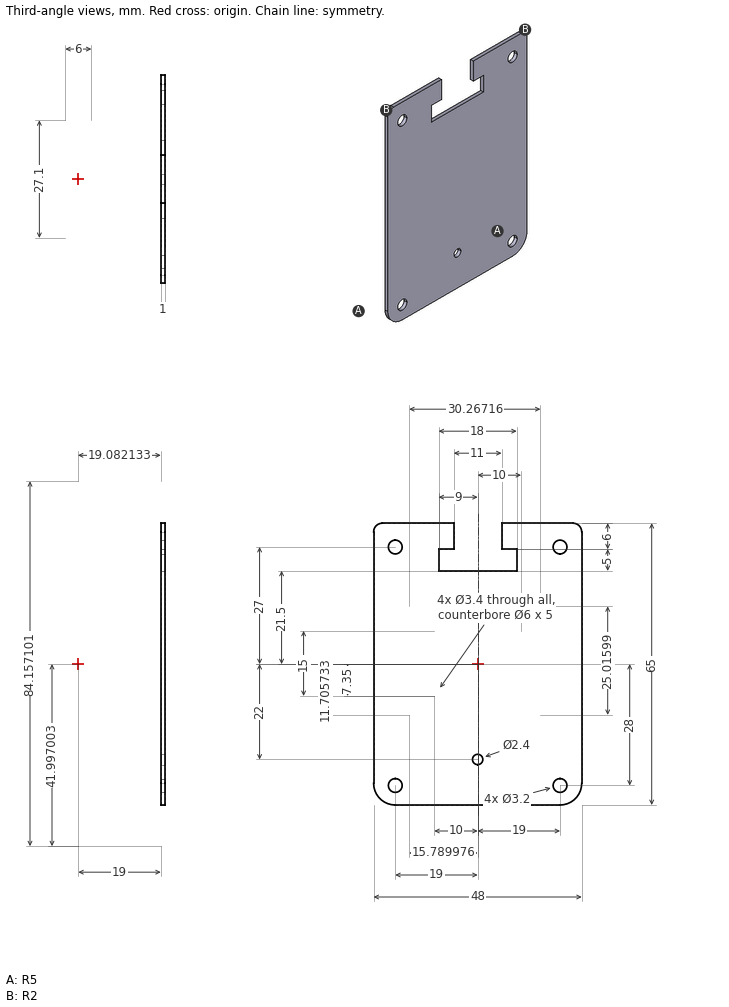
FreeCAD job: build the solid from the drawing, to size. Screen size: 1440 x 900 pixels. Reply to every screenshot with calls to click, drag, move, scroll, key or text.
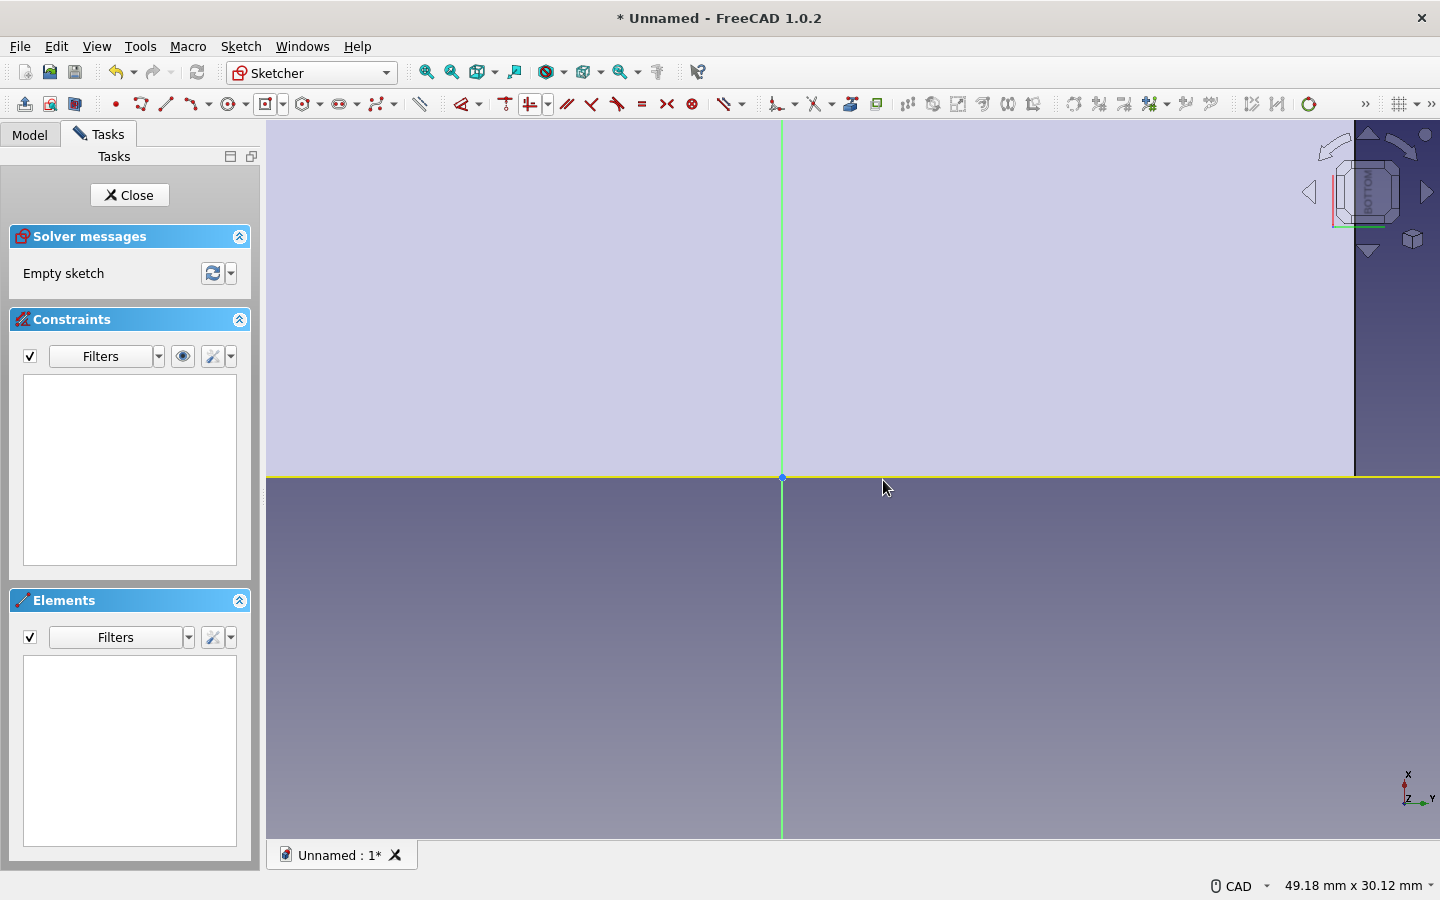
click(264, 104)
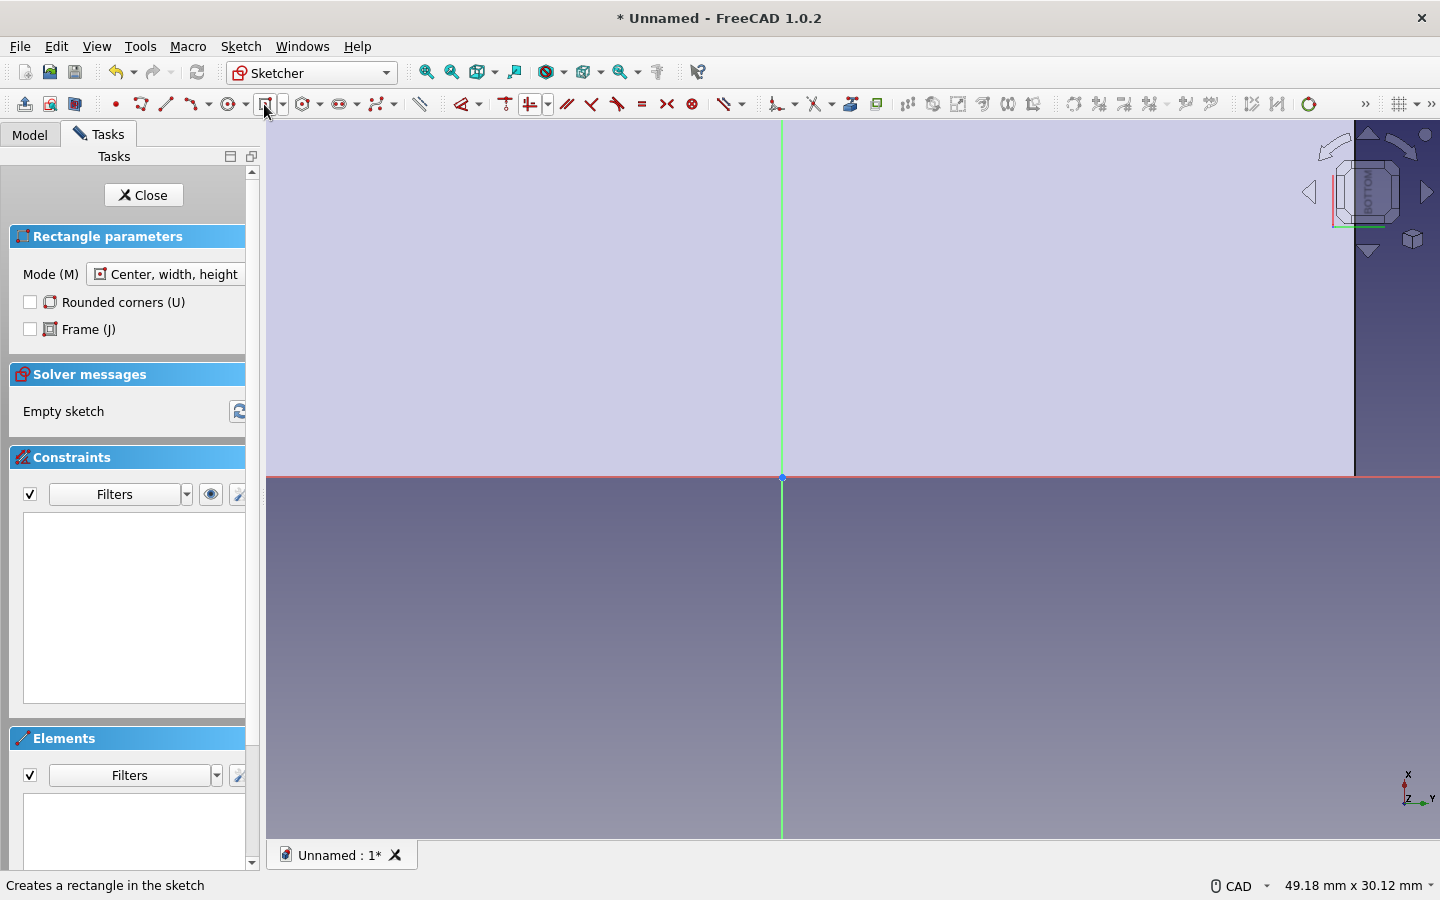
click(782, 477)
move(1106, 406)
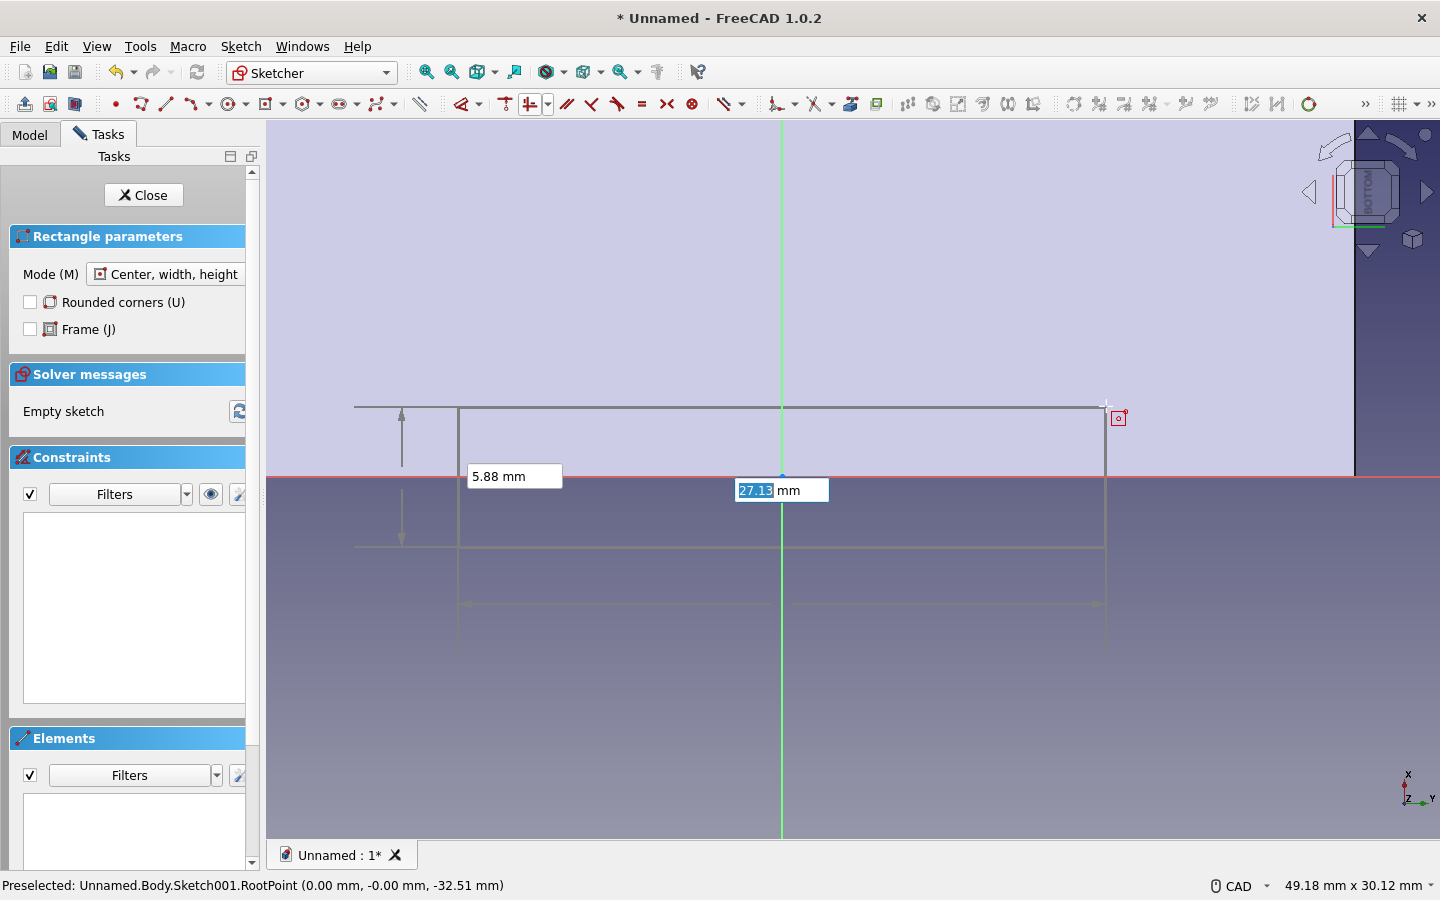
text(27.1)
key(Tab)
text(6)
key(Return)
key(Escape)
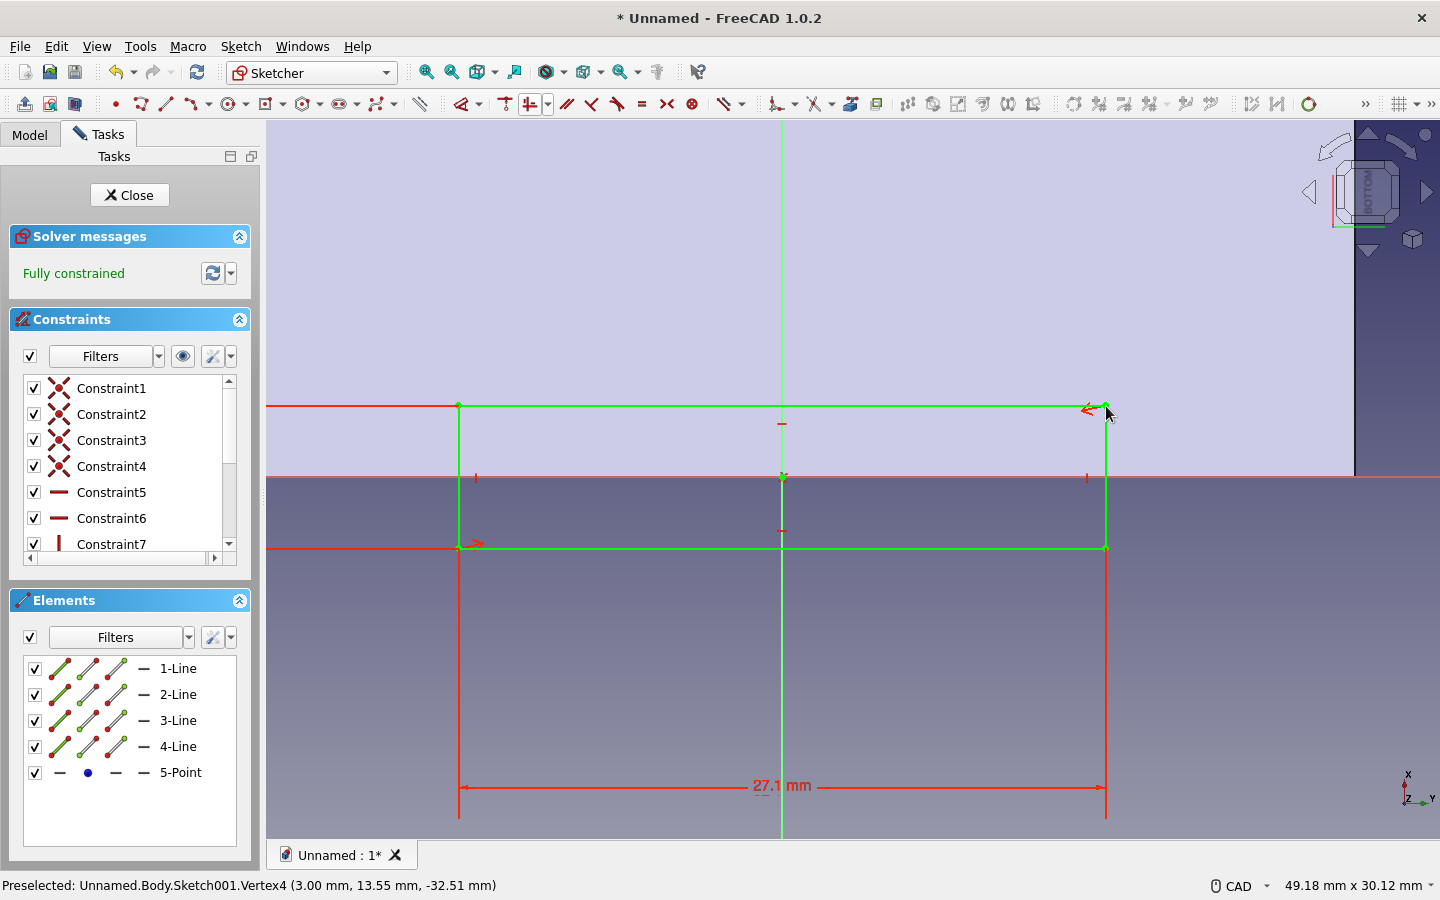
click(130, 195)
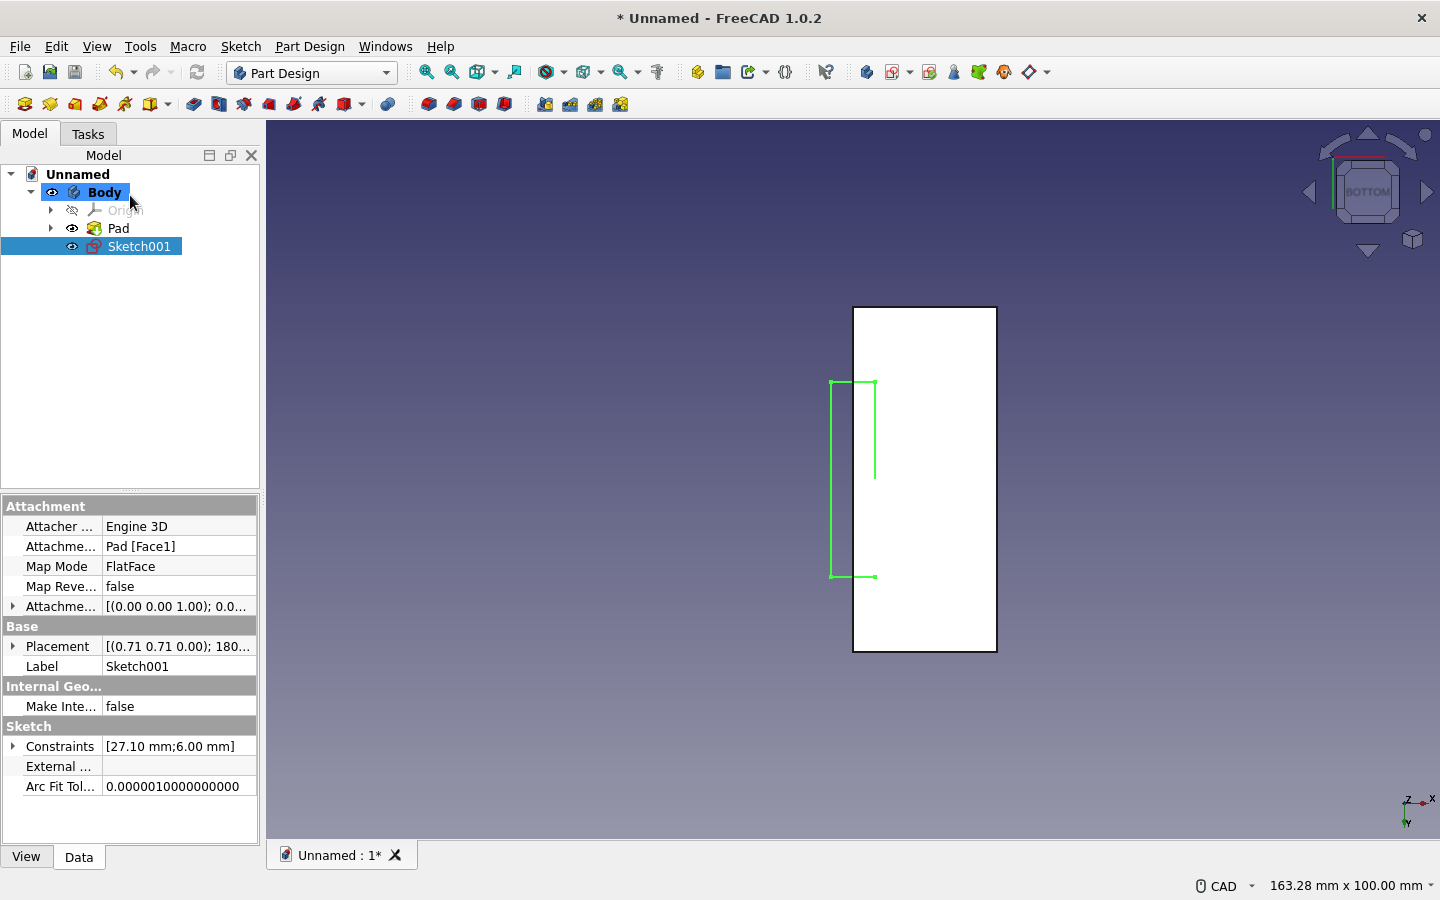
click(194, 104)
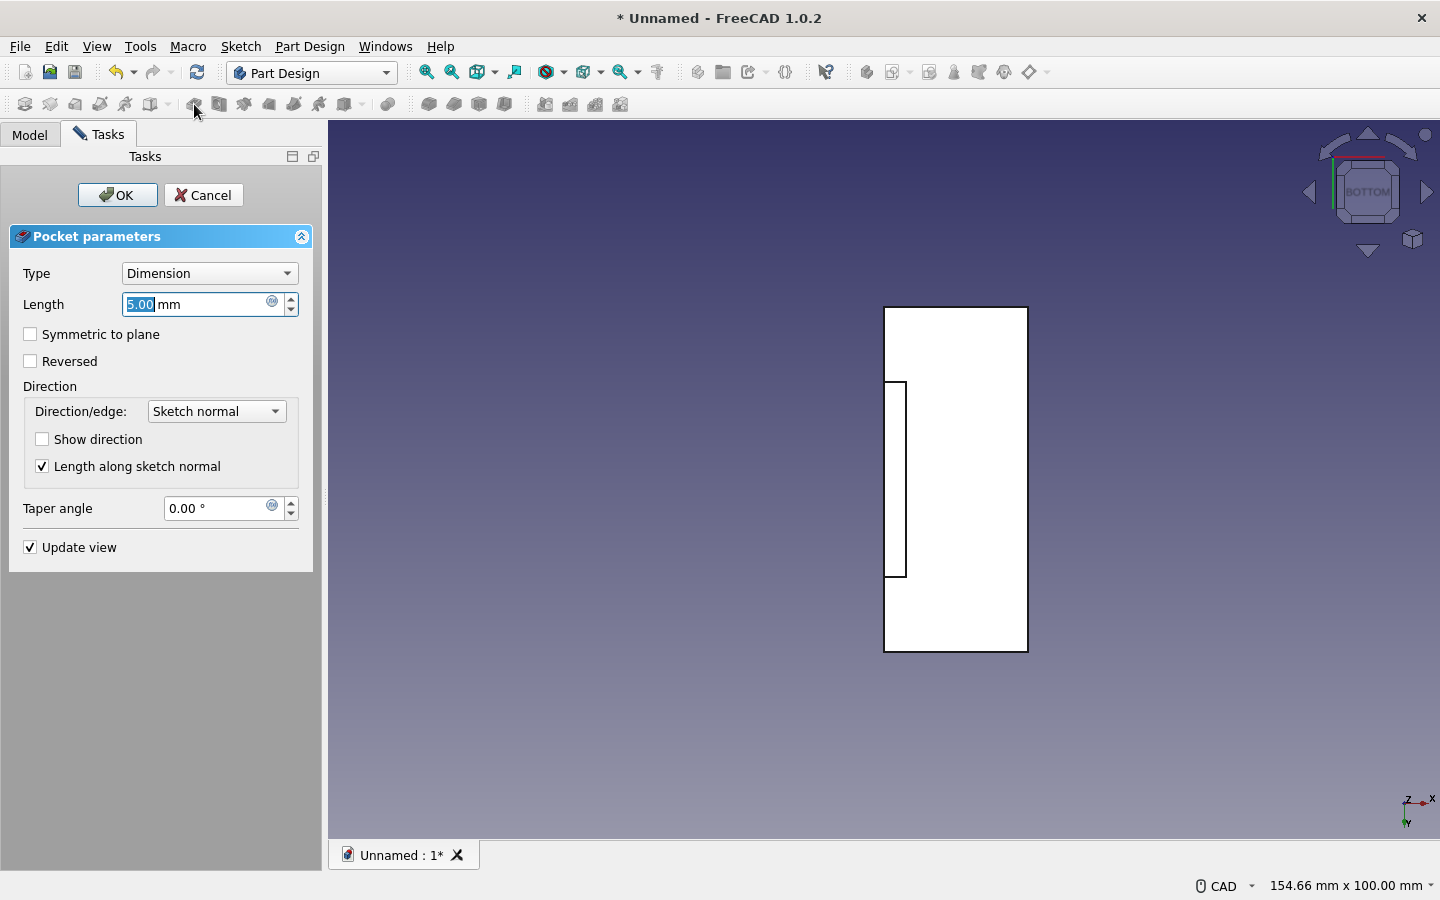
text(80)
key(Tab)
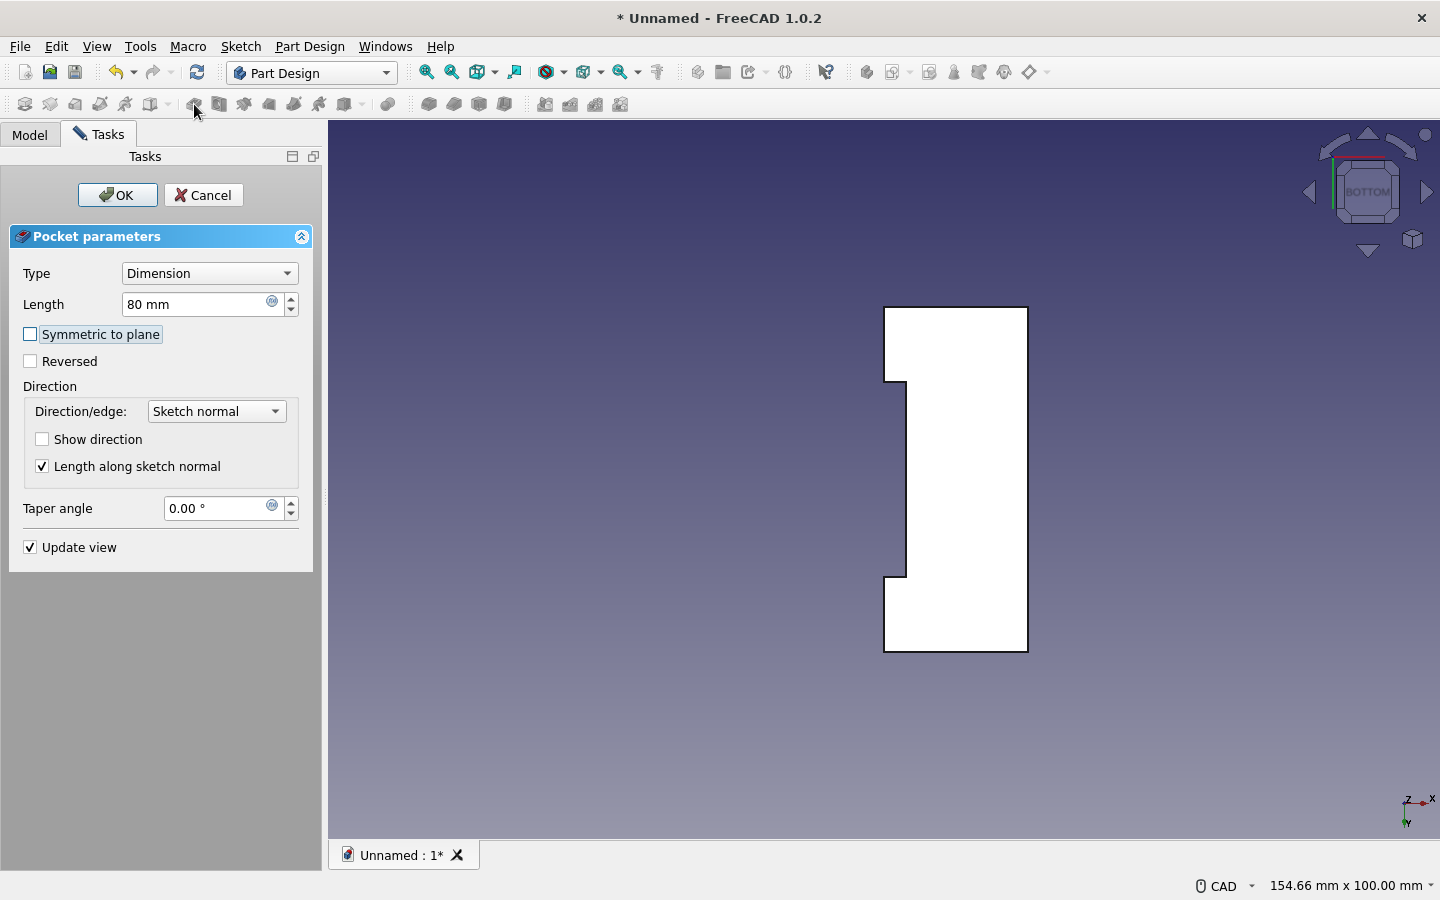
click(118, 195)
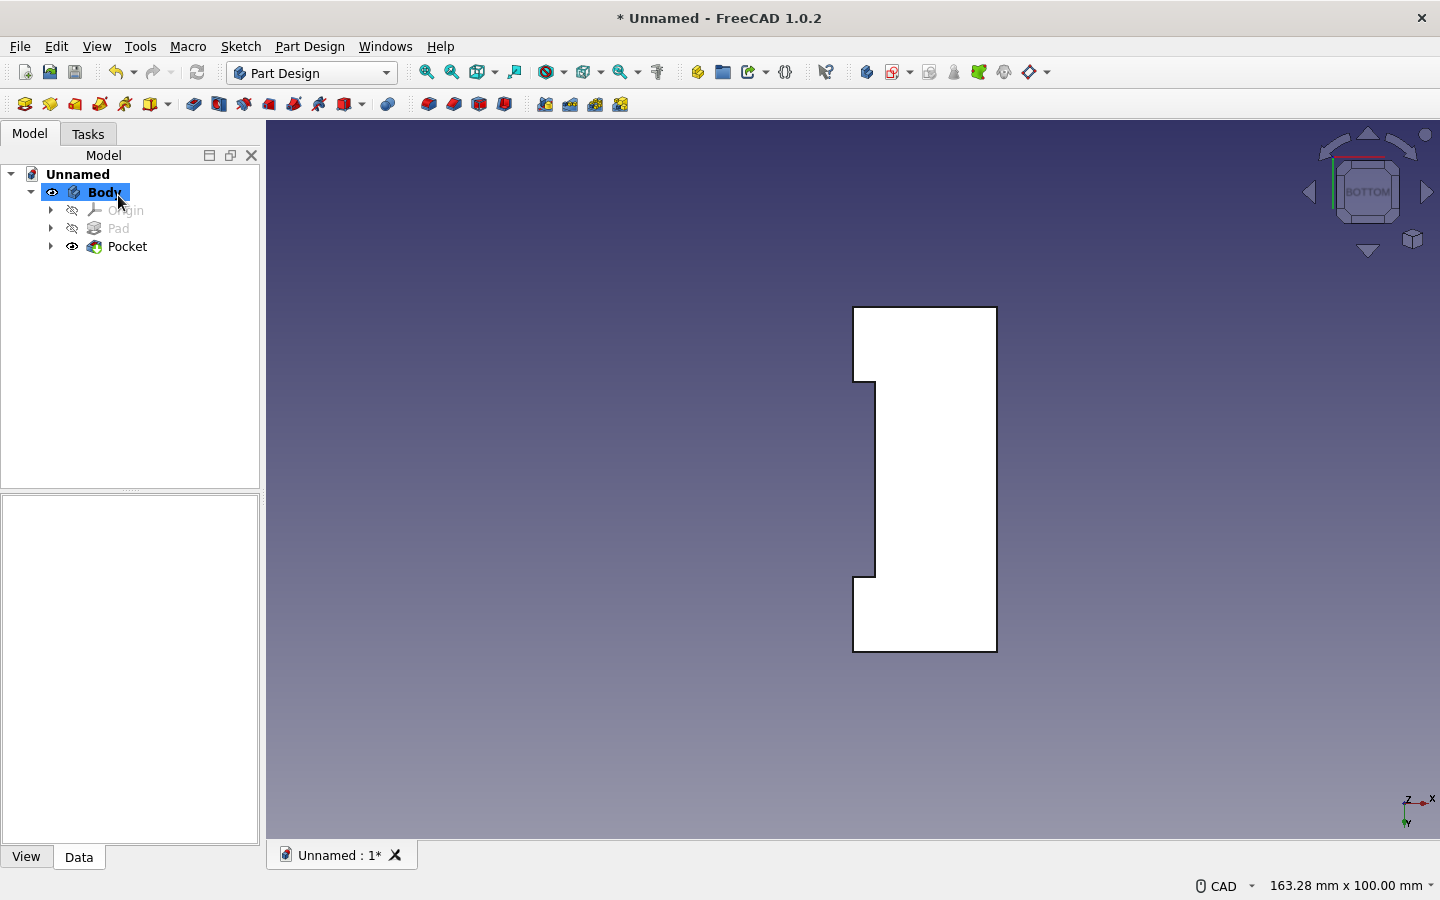
key(0)